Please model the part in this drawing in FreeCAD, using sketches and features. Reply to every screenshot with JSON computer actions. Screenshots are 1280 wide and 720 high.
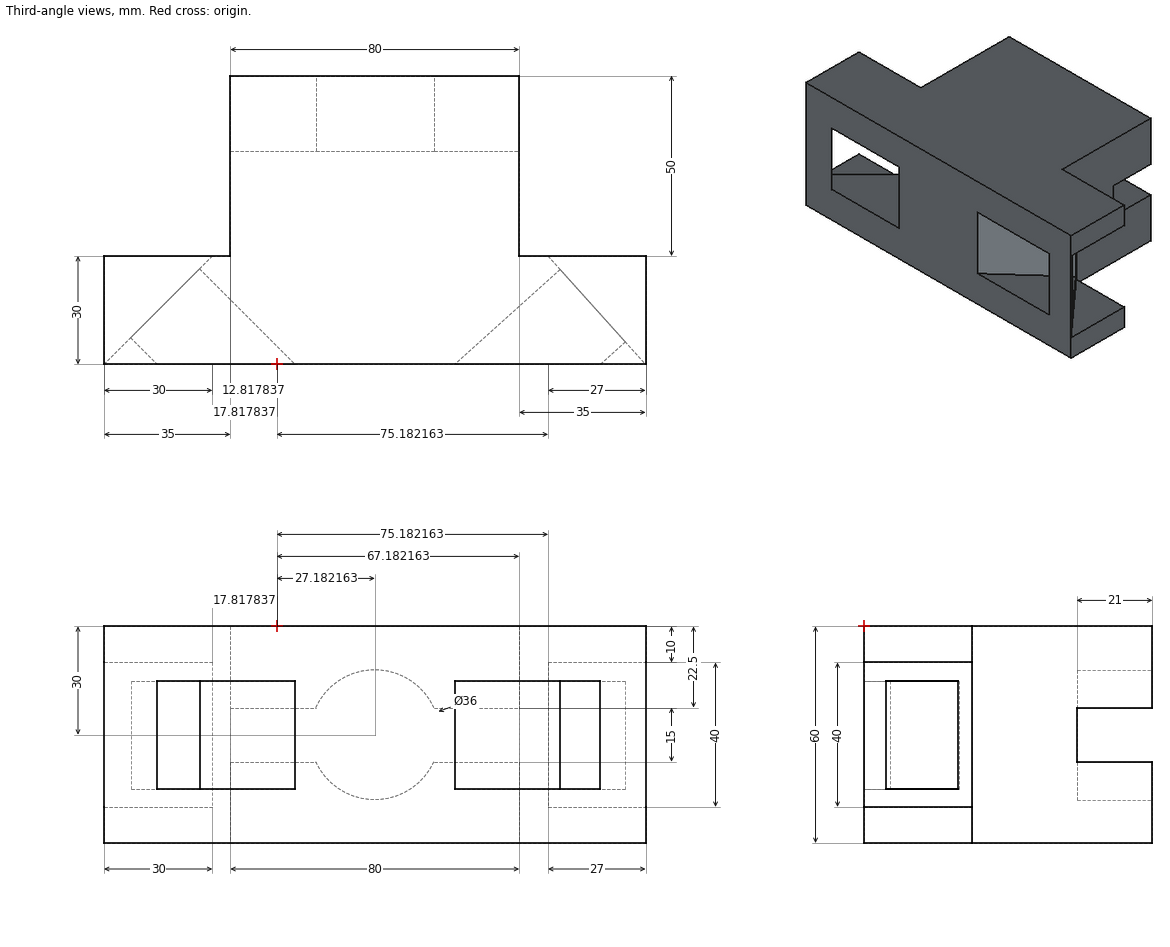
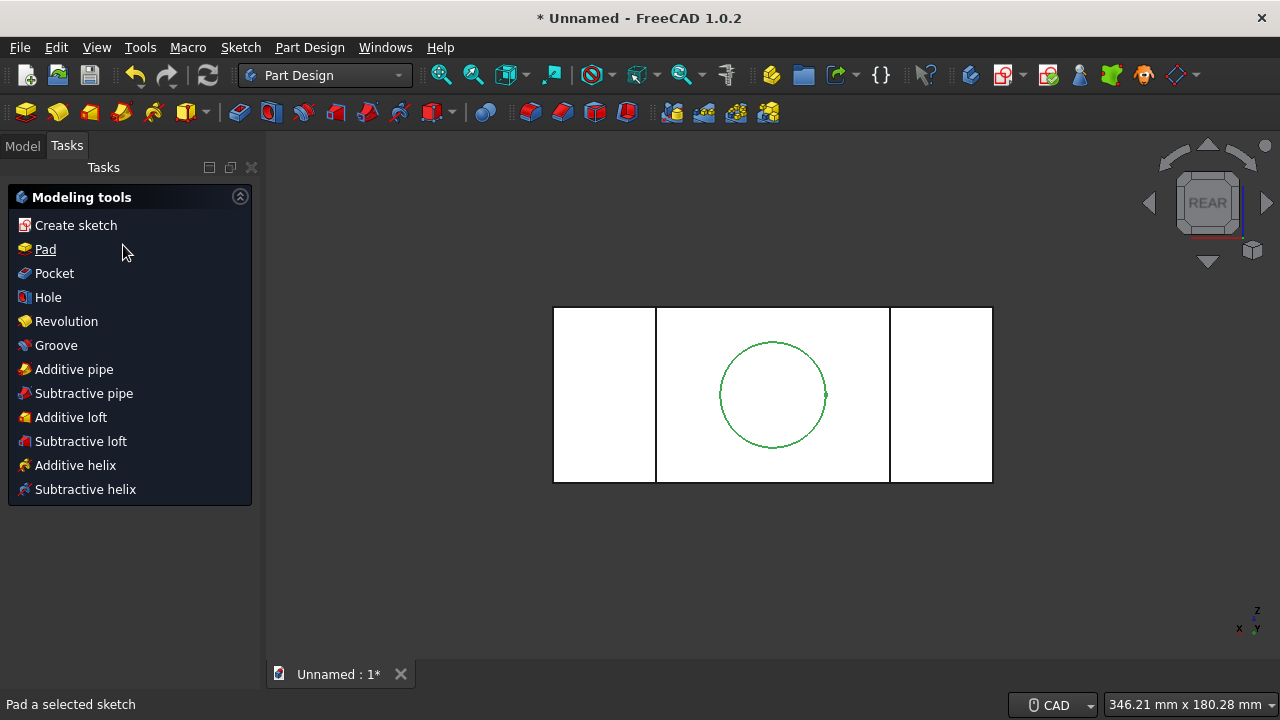
{"action": "left_click", "coordinate": [240, 112]}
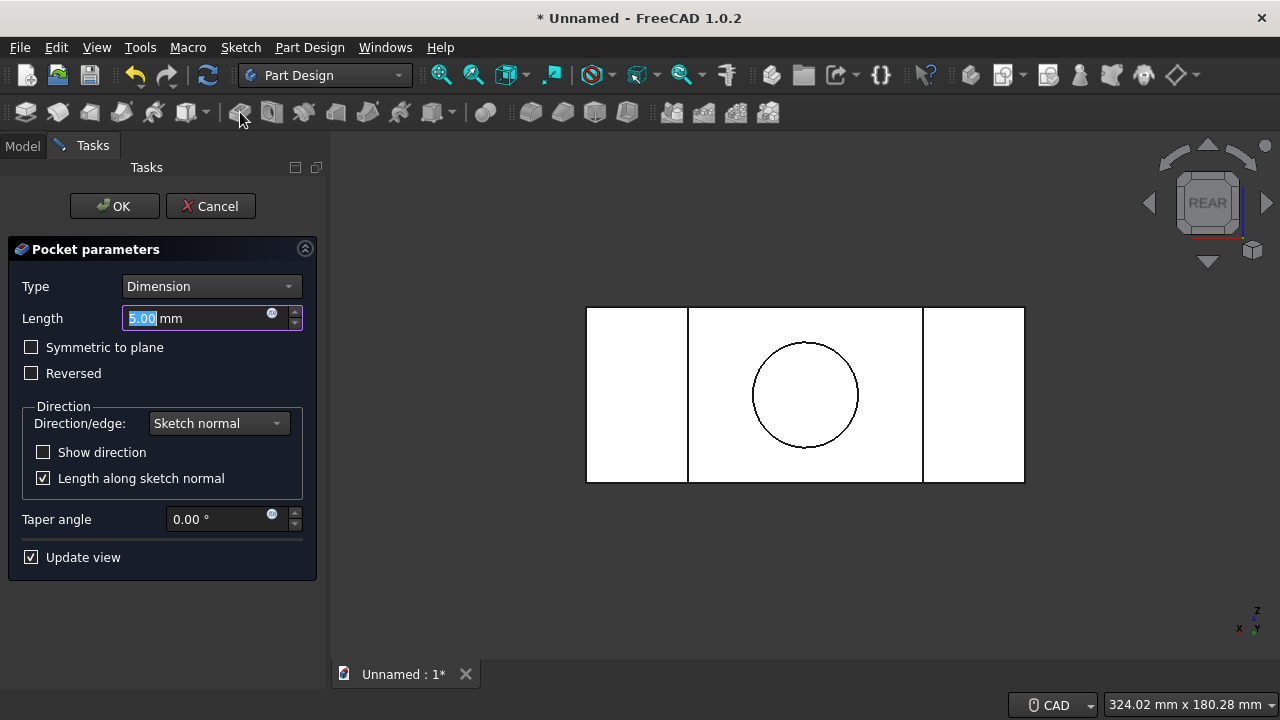
{"action": "type", "text": "21"}
{"action": "key", "text": "Tab"}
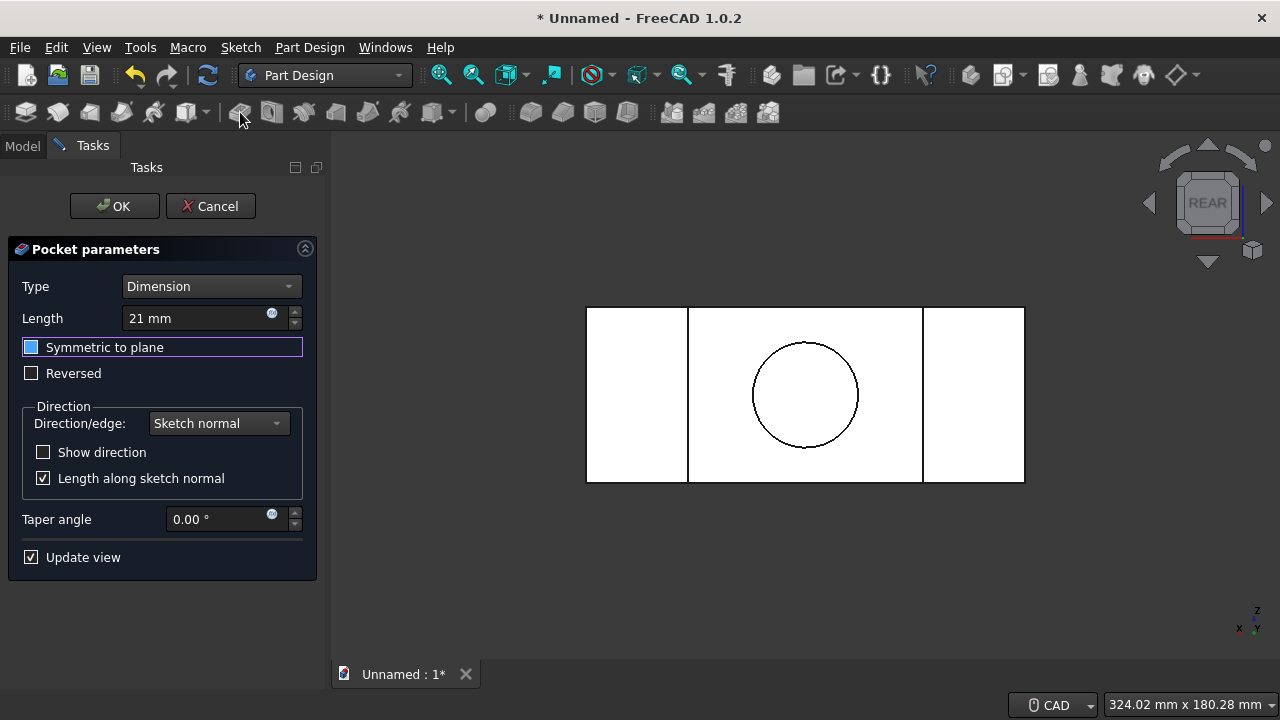
{"action": "left_click", "coordinate": [115, 206]}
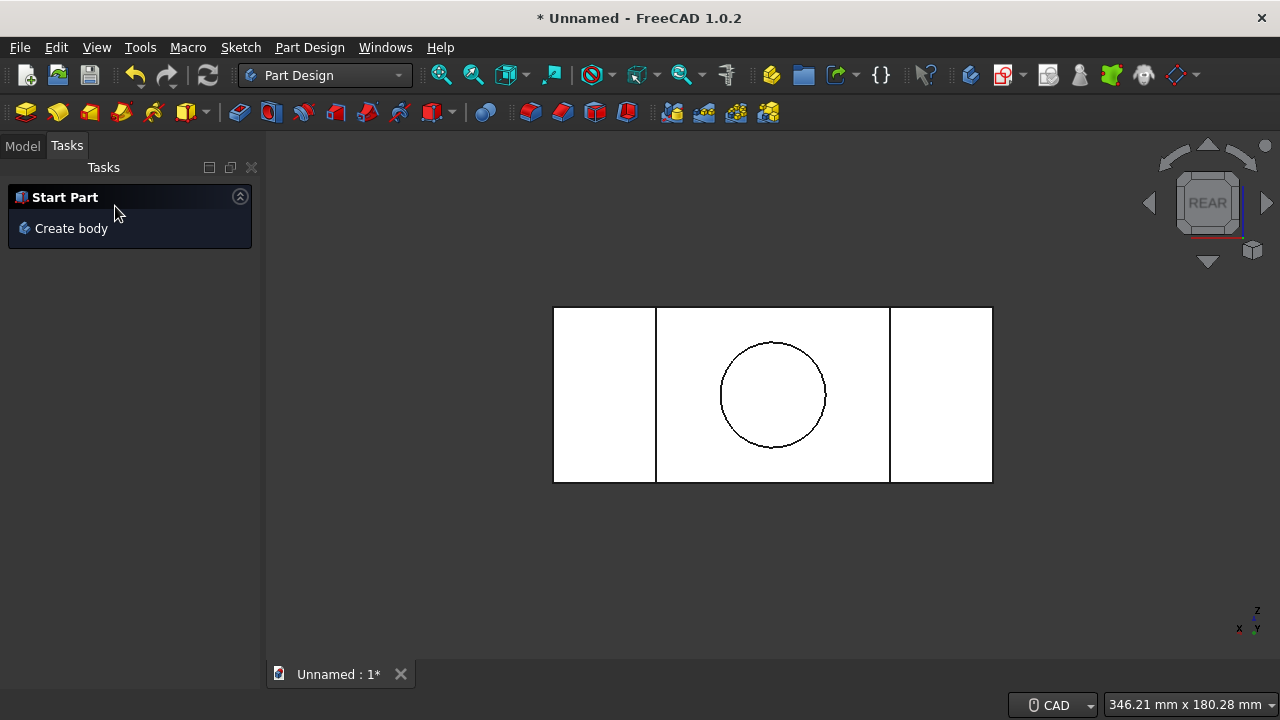
{"action": "left_click", "coordinate": [442, 76]}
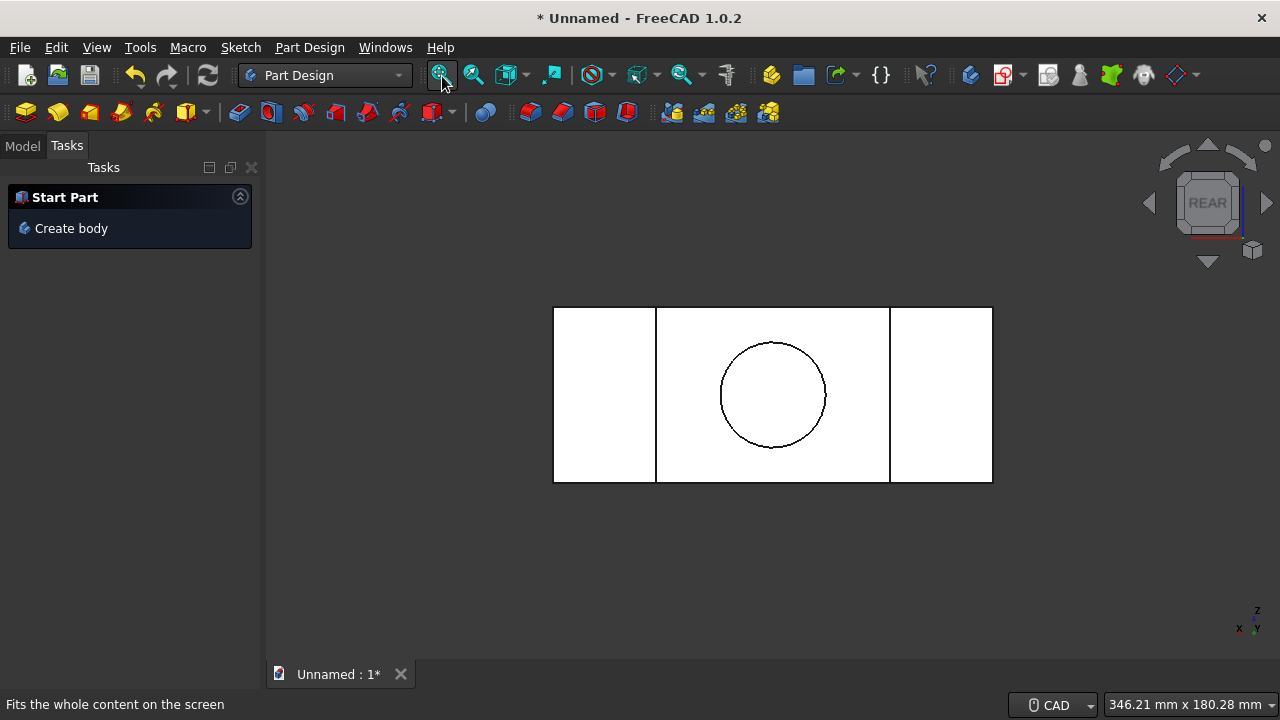
{"action": "left_click", "coordinate": [706, 344]}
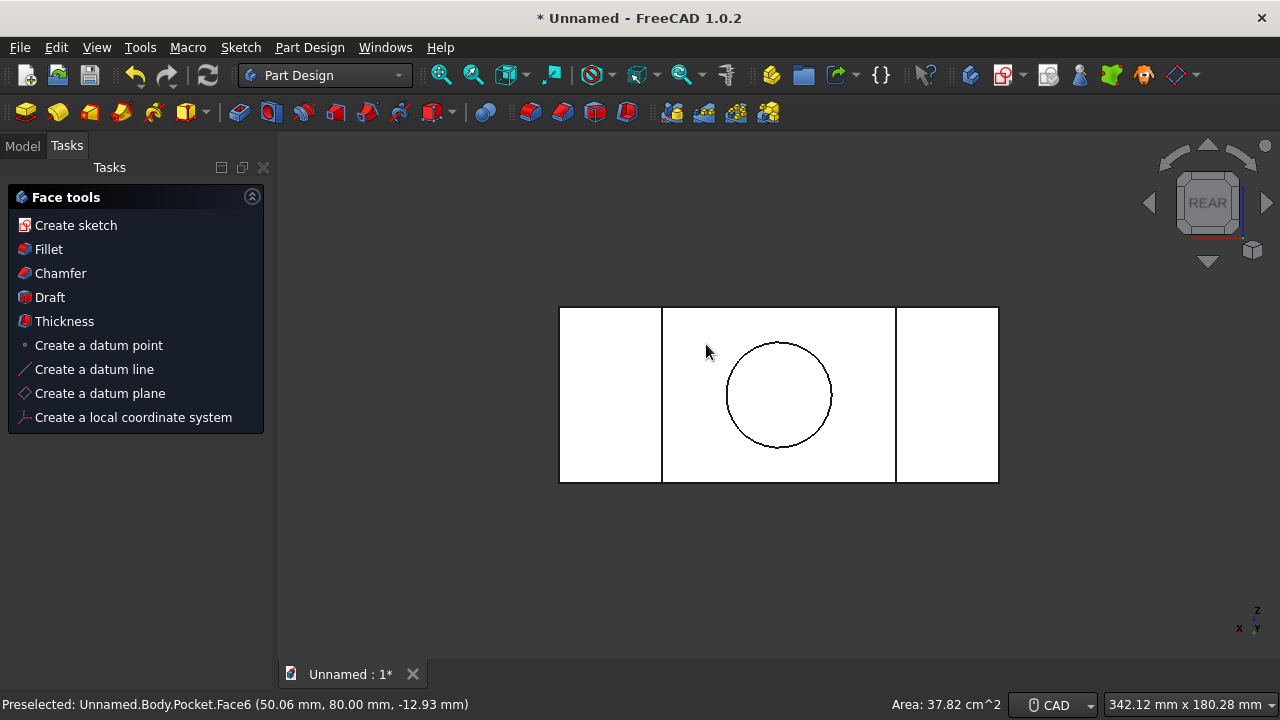
{"action": "left_click", "coordinate": [1004, 76]}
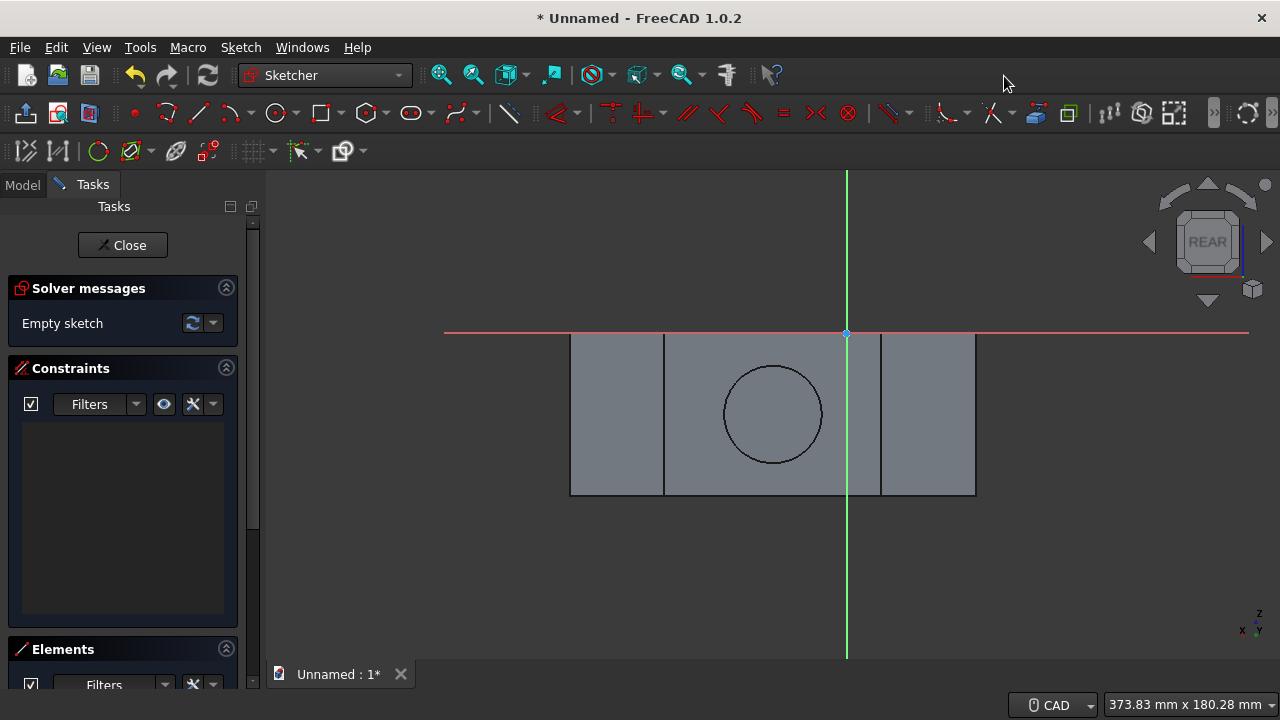
{"action": "scroll", "coordinate": [813, 366], "scroll_direction": "up", "scroll_amount": 5}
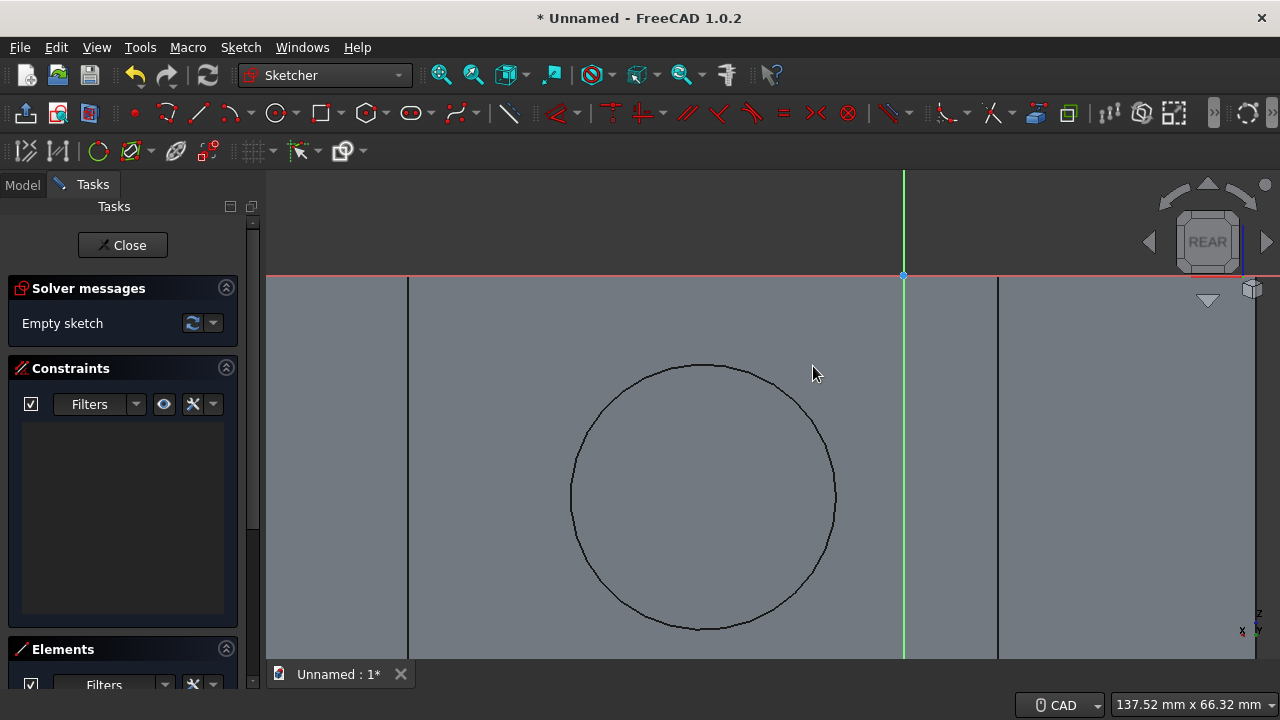
{"action": "left_click", "coordinate": [322, 114]}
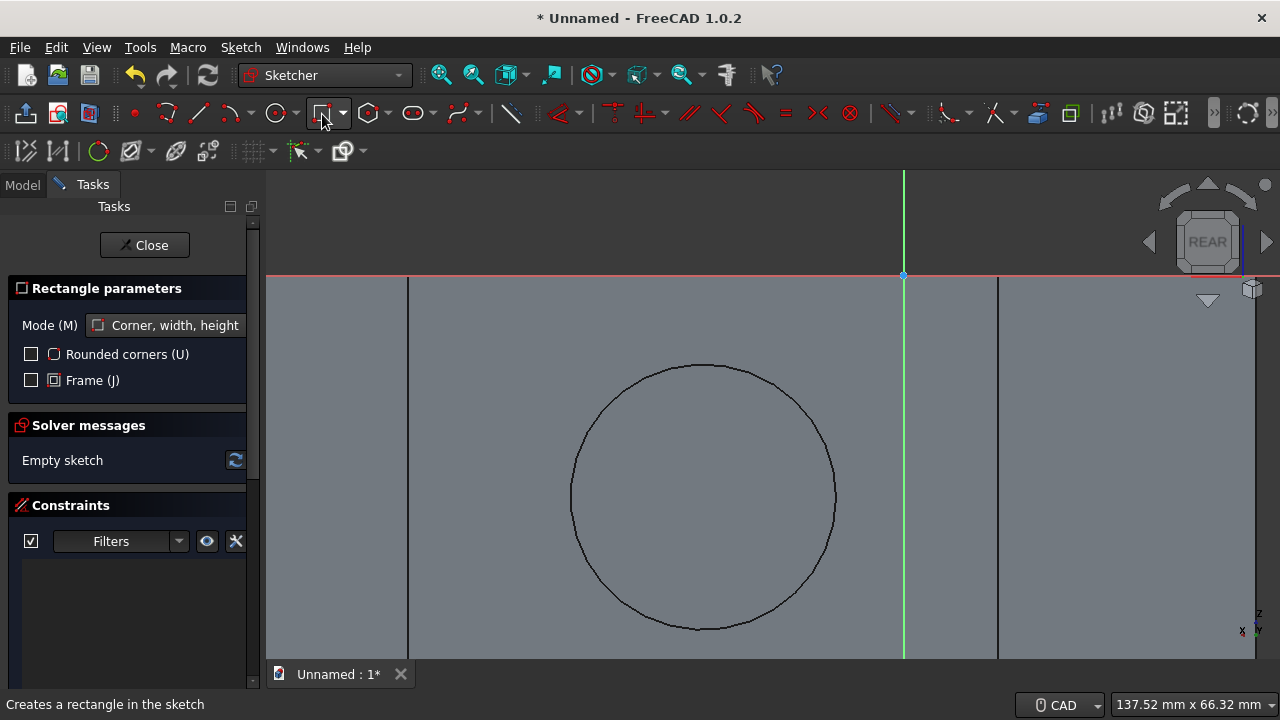
{"action": "left_click", "coordinate": [408, 442]}
{"action": "left_click", "coordinate": [998, 552]}
{"action": "key", "text": "Escape"}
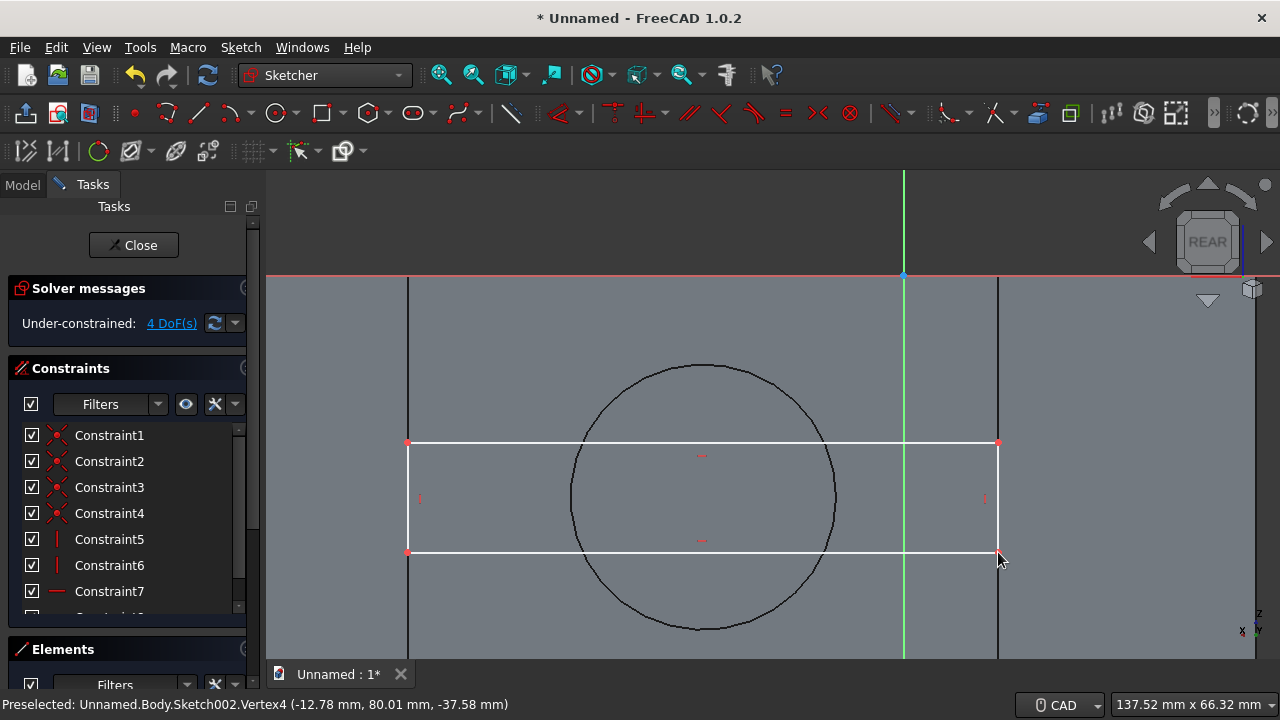
{"action": "left_click", "coordinate": [558, 114]}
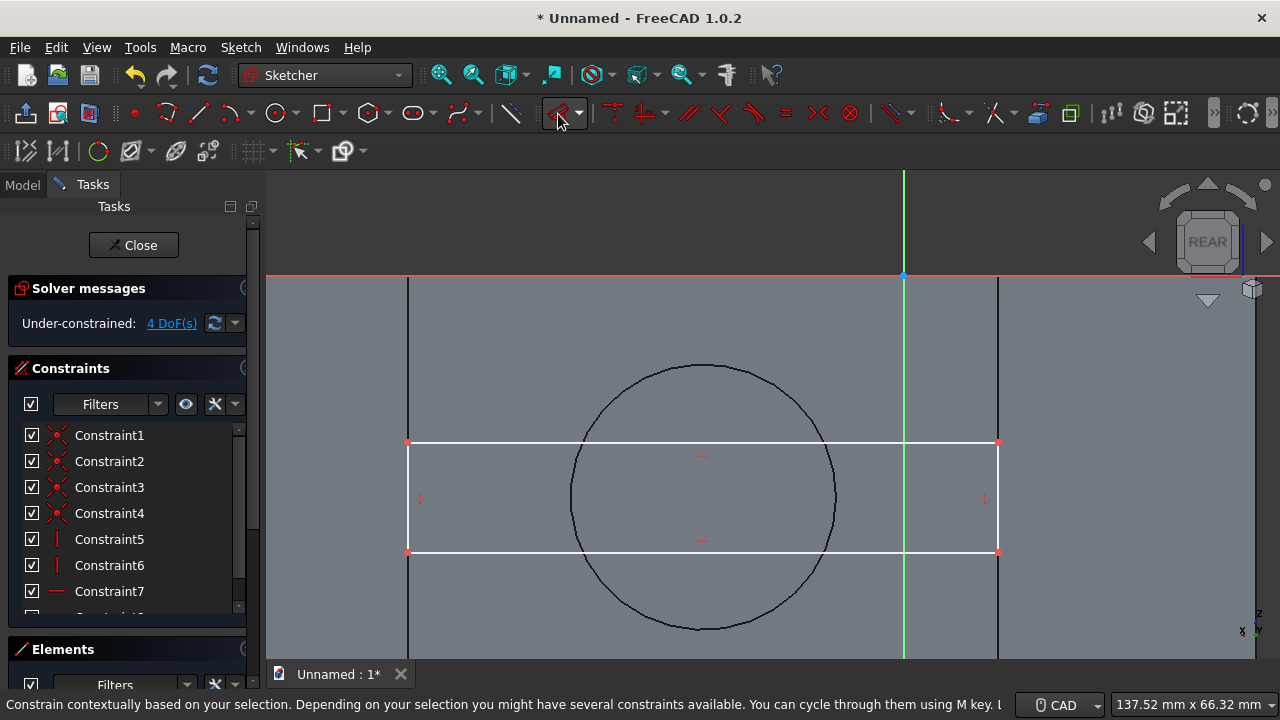
{"action": "left_click", "coordinate": [408, 476]}
{"action": "left_click", "coordinate": [374, 498]}